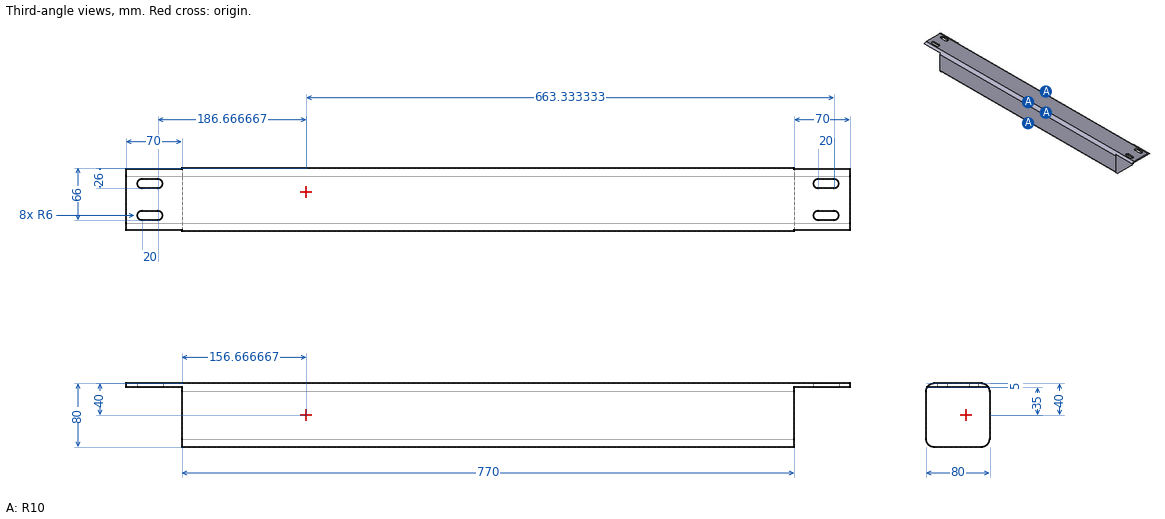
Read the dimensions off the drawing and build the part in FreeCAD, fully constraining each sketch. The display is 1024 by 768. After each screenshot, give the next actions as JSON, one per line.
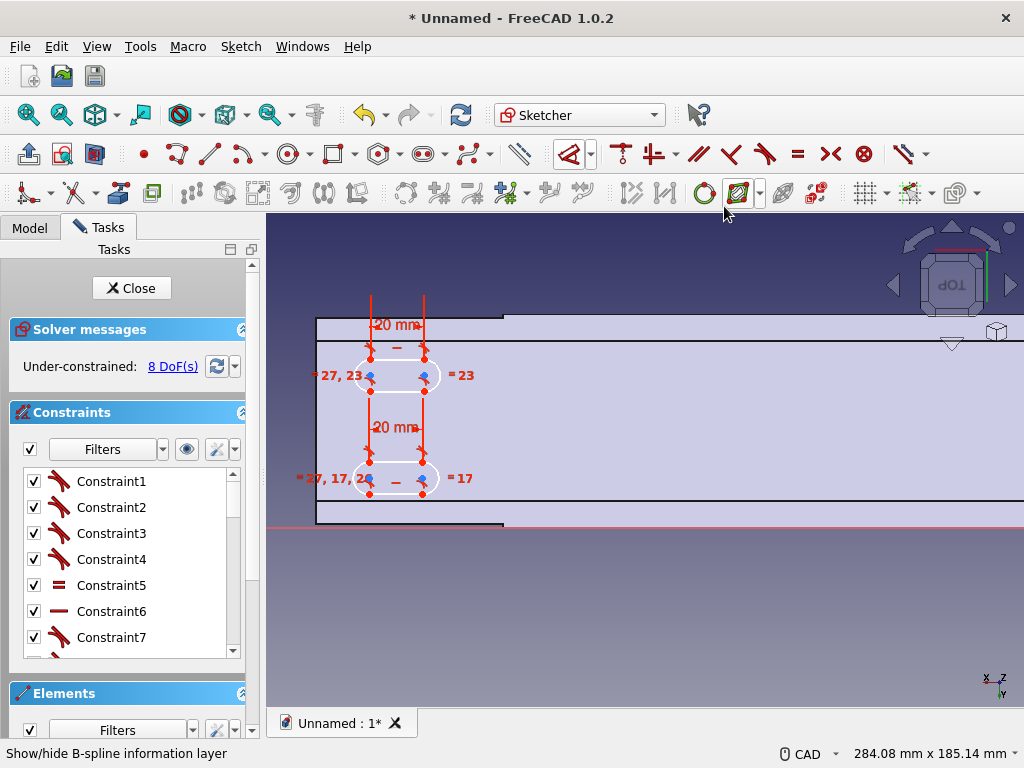
{"action": "scroll", "coordinate": [388, 464], "scroll_direction": "down", "scroll_amount": 9}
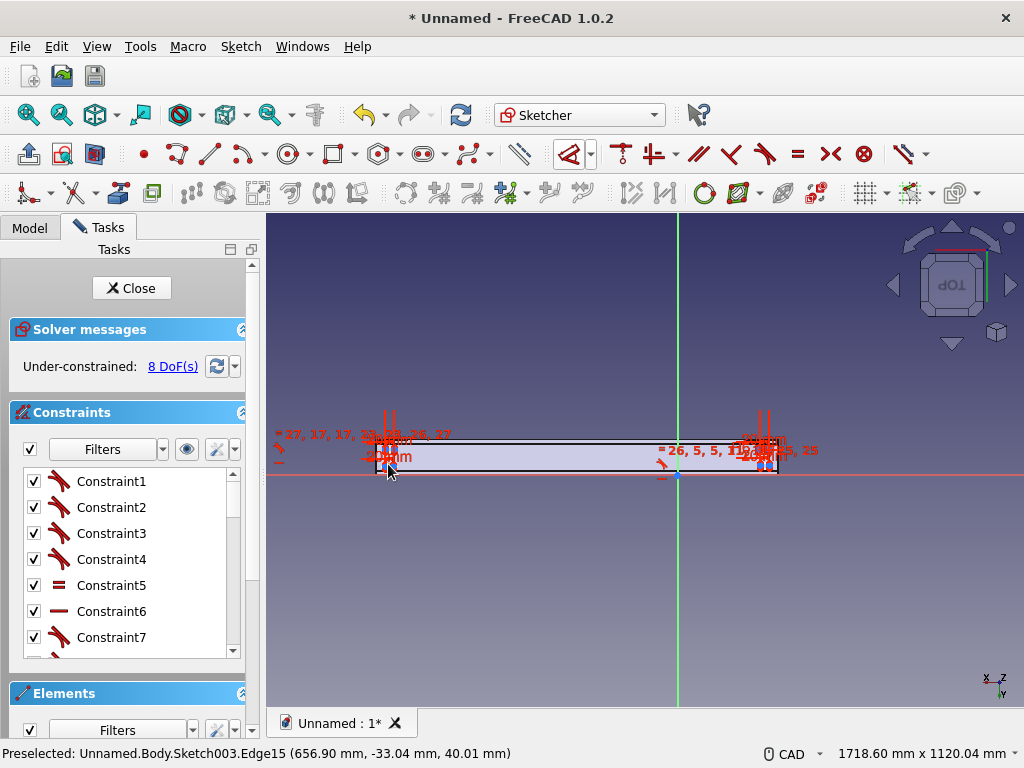
{"action": "scroll", "coordinate": [760, 447], "scroll_direction": "up", "scroll_amount": 8}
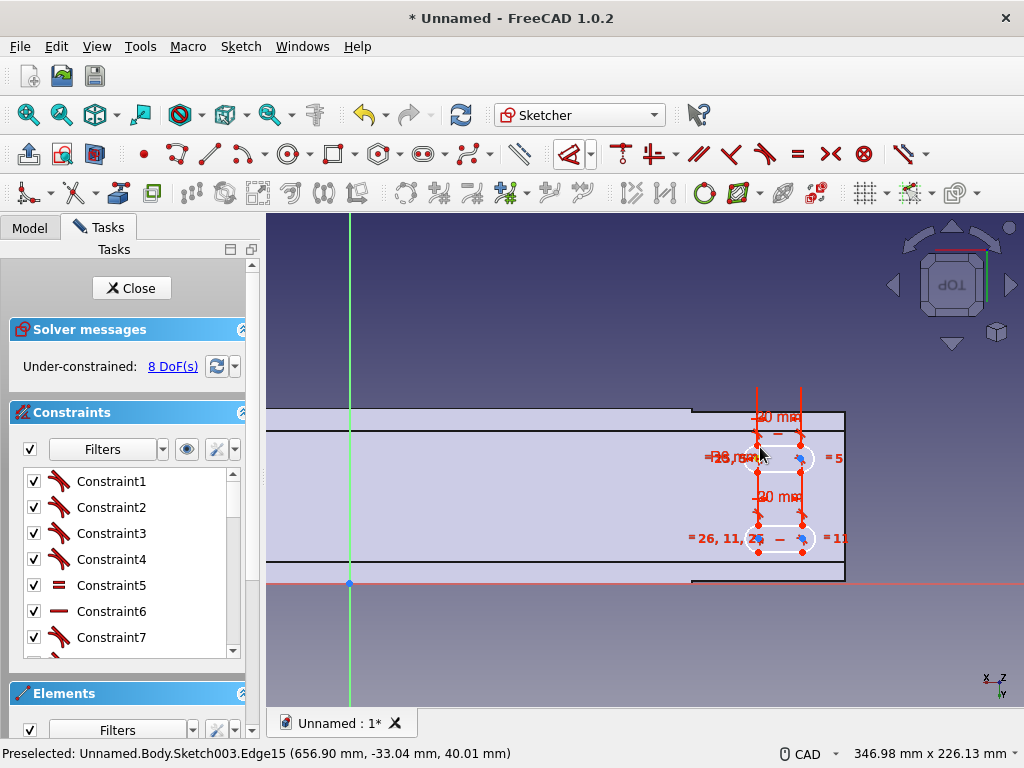
{"action": "left_click", "coordinate": [757, 446]}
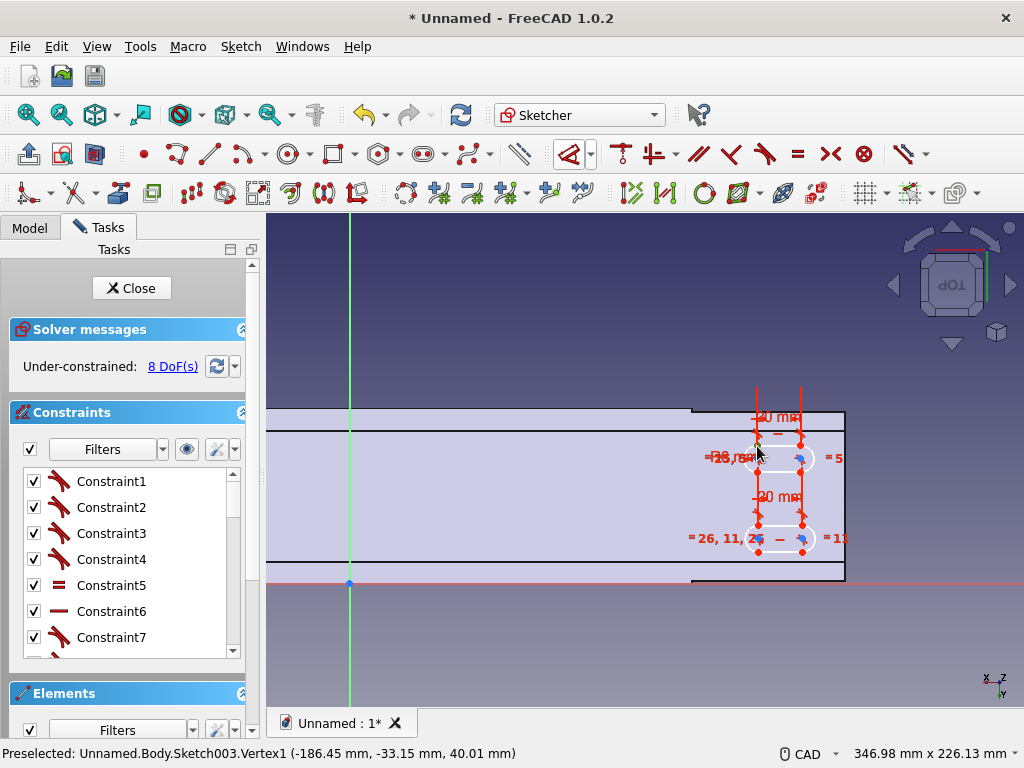
{"action": "key", "text": "i"}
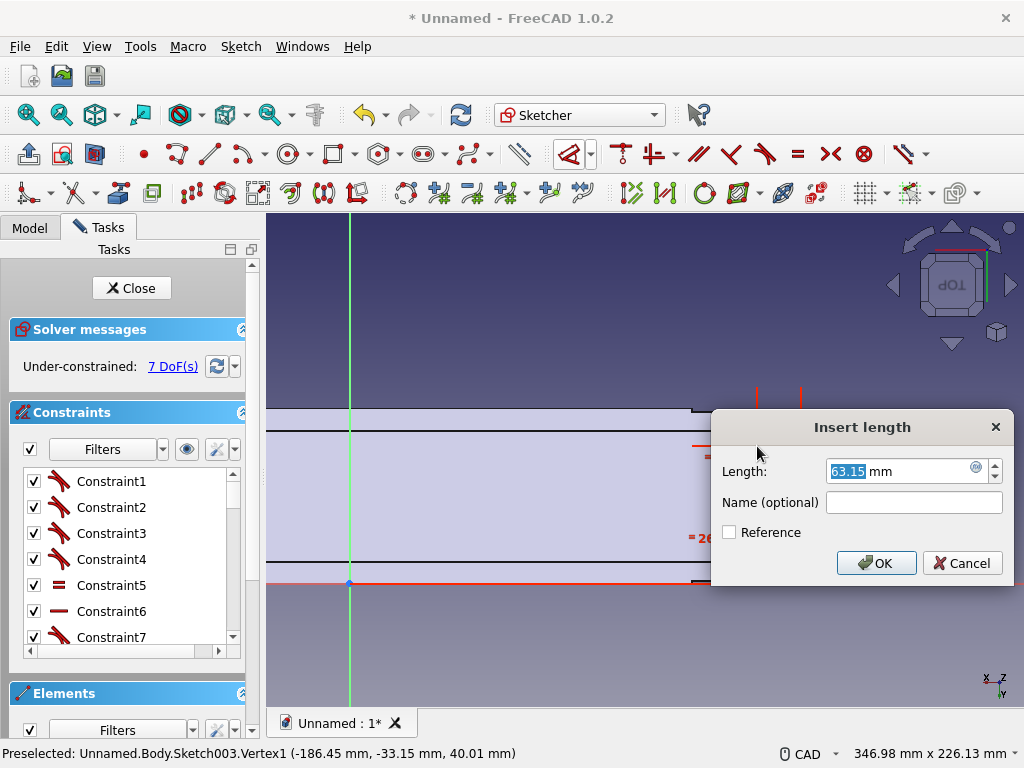
{"action": "type", "text": "66"}
{"action": "key", "text": "Return"}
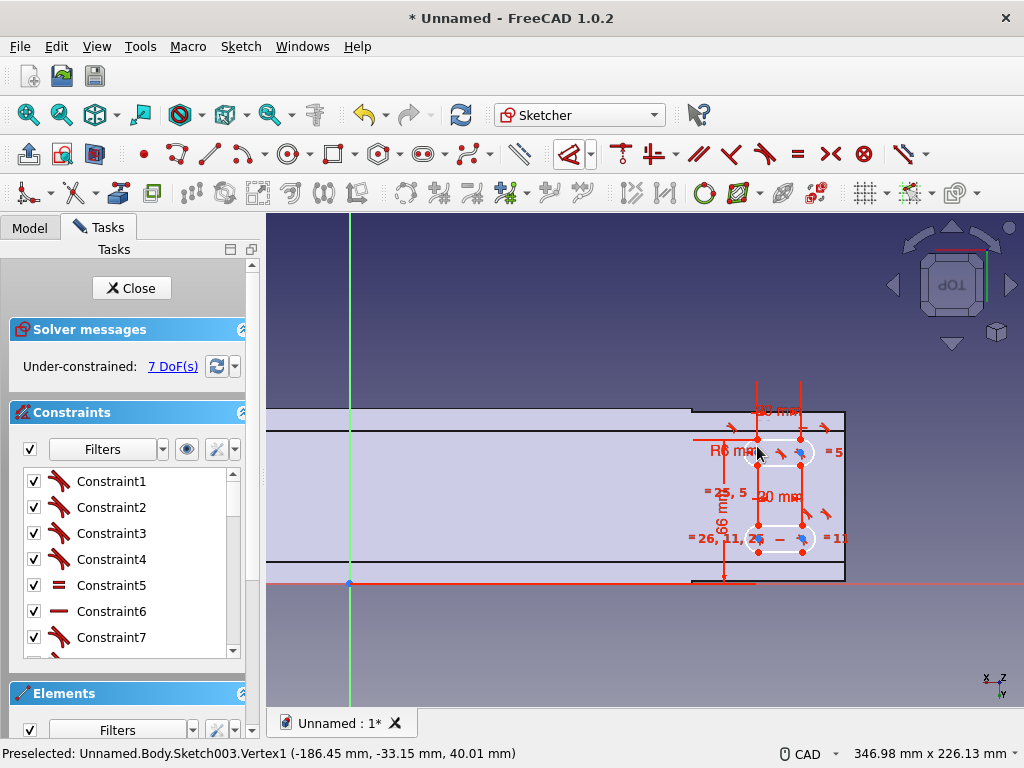
{"action": "left_click", "coordinate": [758, 526]}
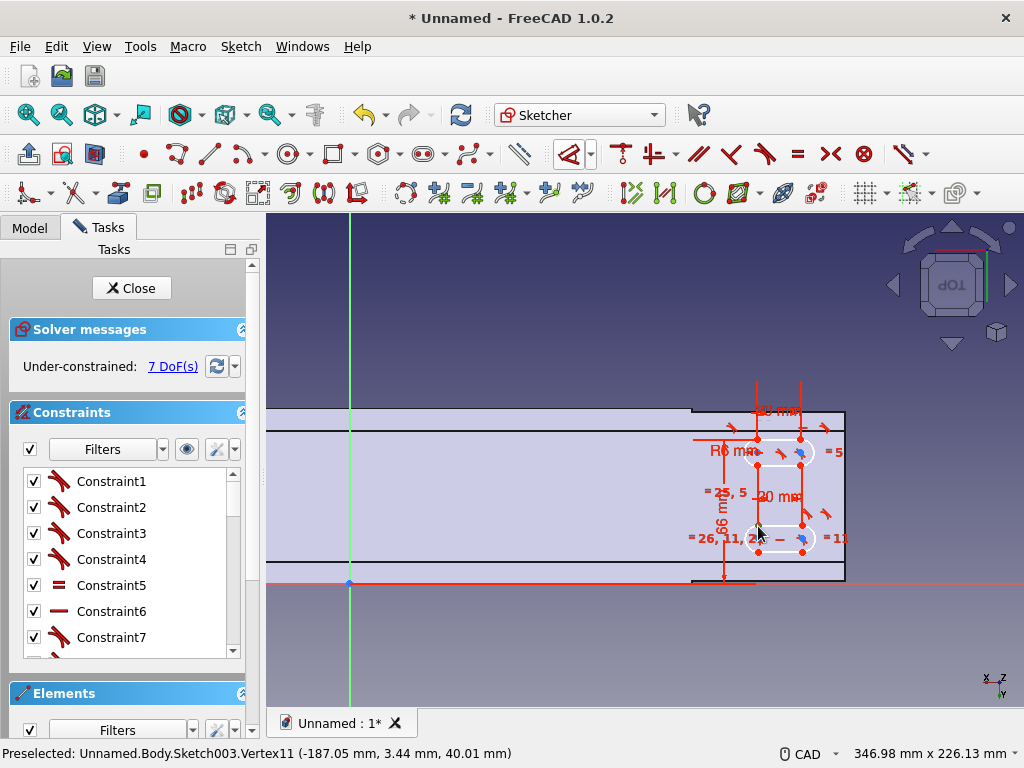
{"action": "left_click", "coordinate": [590, 154]}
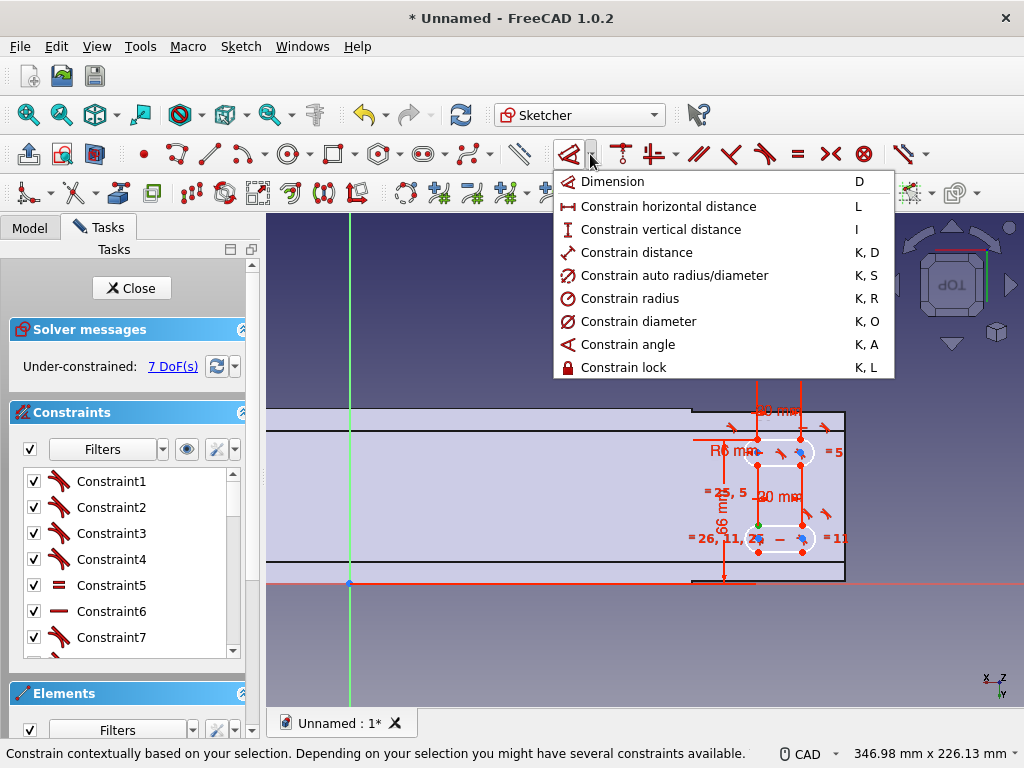
{"action": "left_click", "coordinate": [724, 230]}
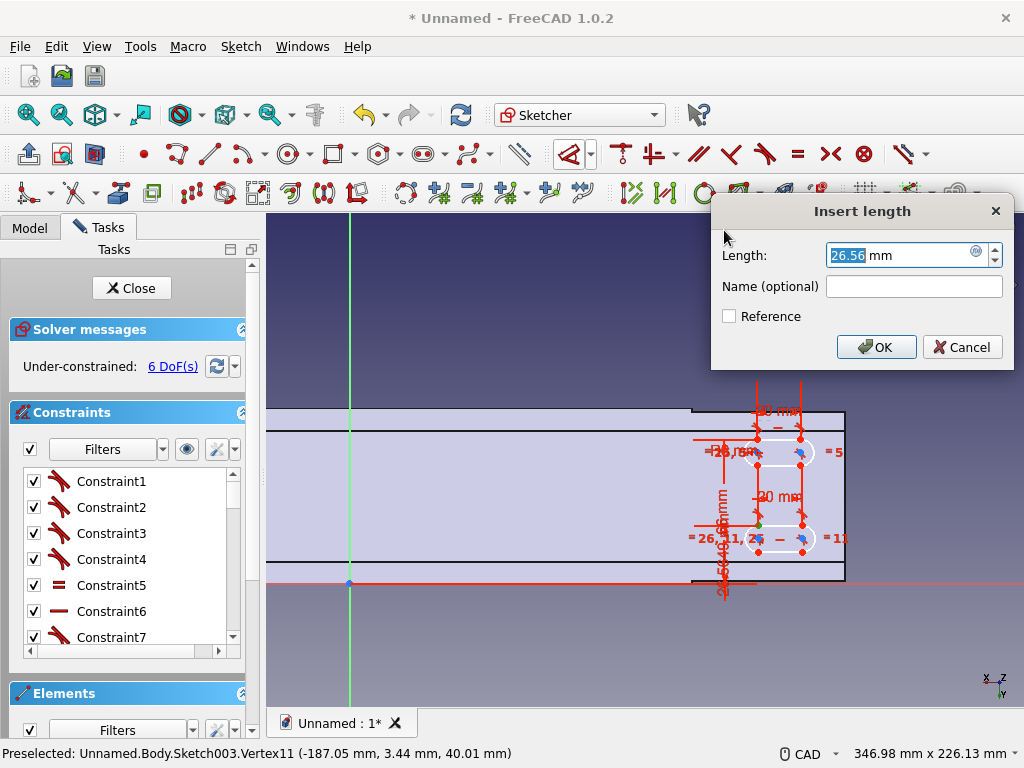
{"action": "type", "text": "26"}
{"action": "key", "text": "Return"}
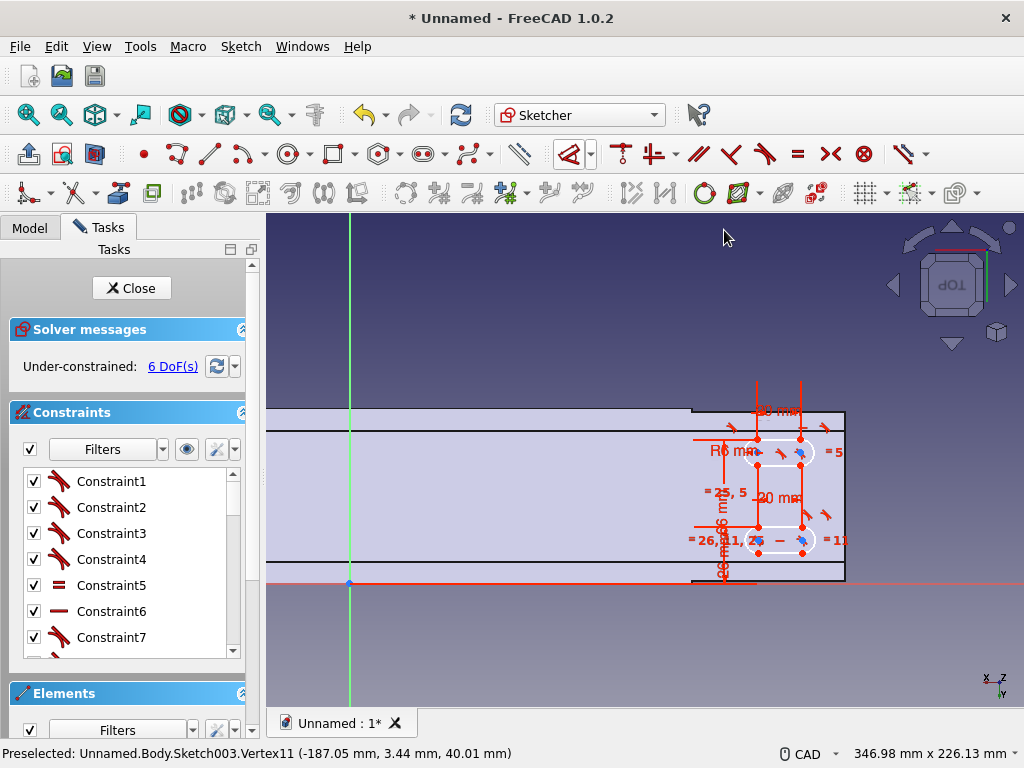
{"action": "scroll", "coordinate": [760, 447], "scroll_direction": "down", "scroll_amount": 8}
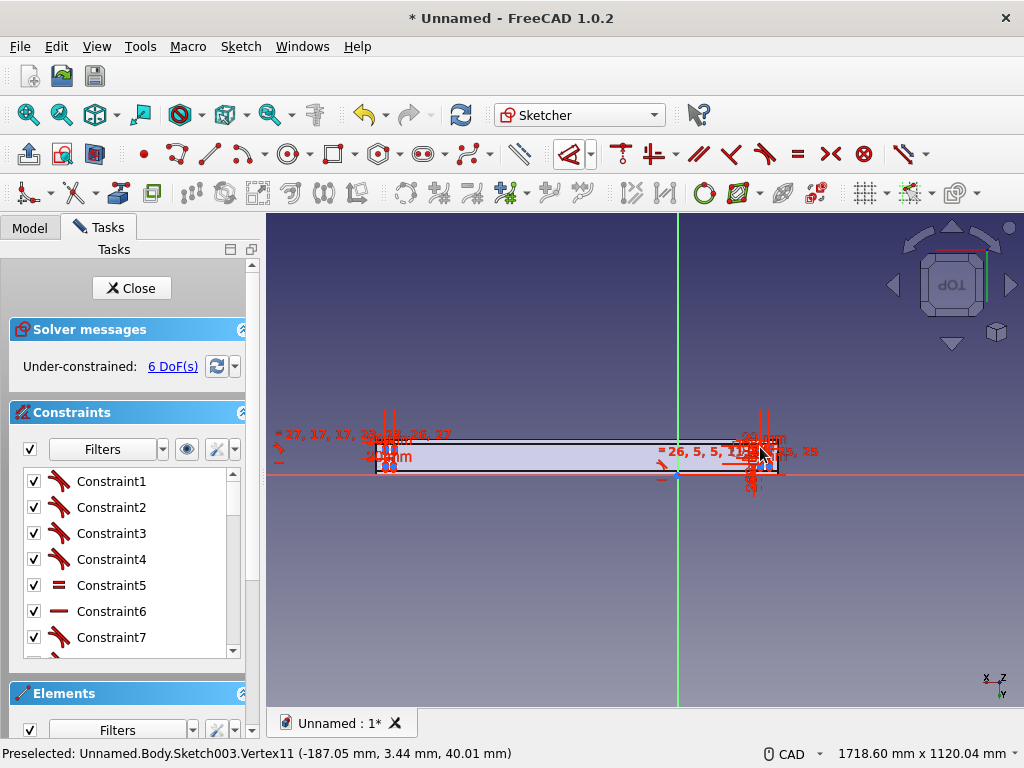
{"action": "scroll", "coordinate": [385, 464], "scroll_direction": "up", "scroll_amount": 8}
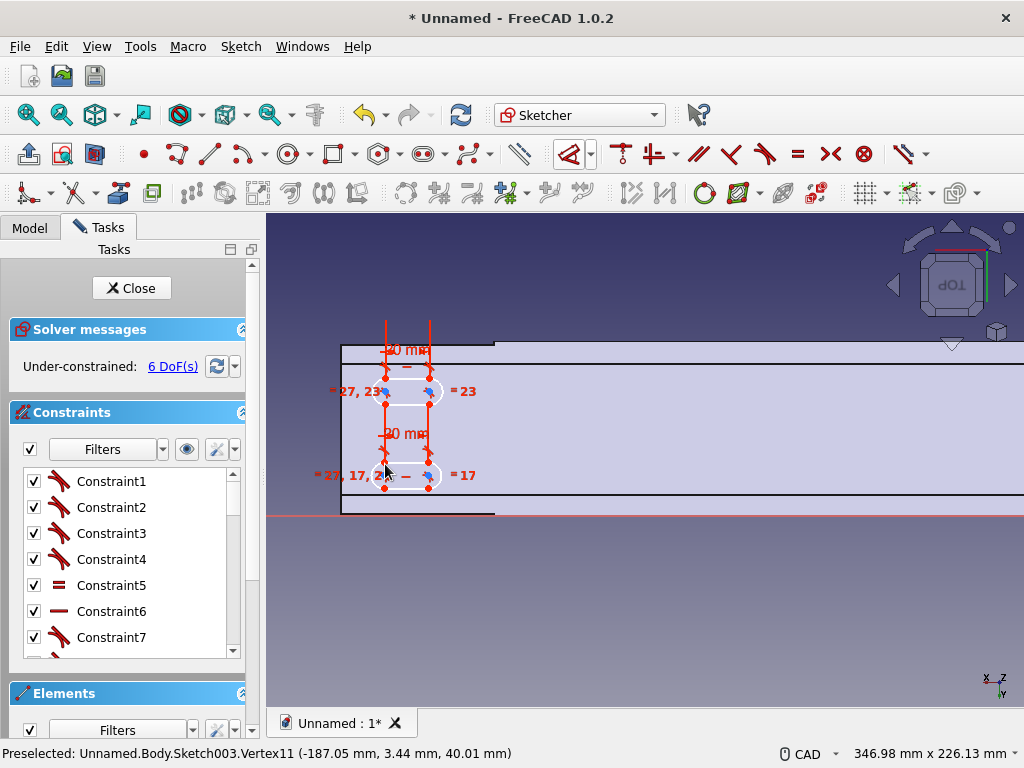
{"action": "left_click", "coordinate": [385, 463]}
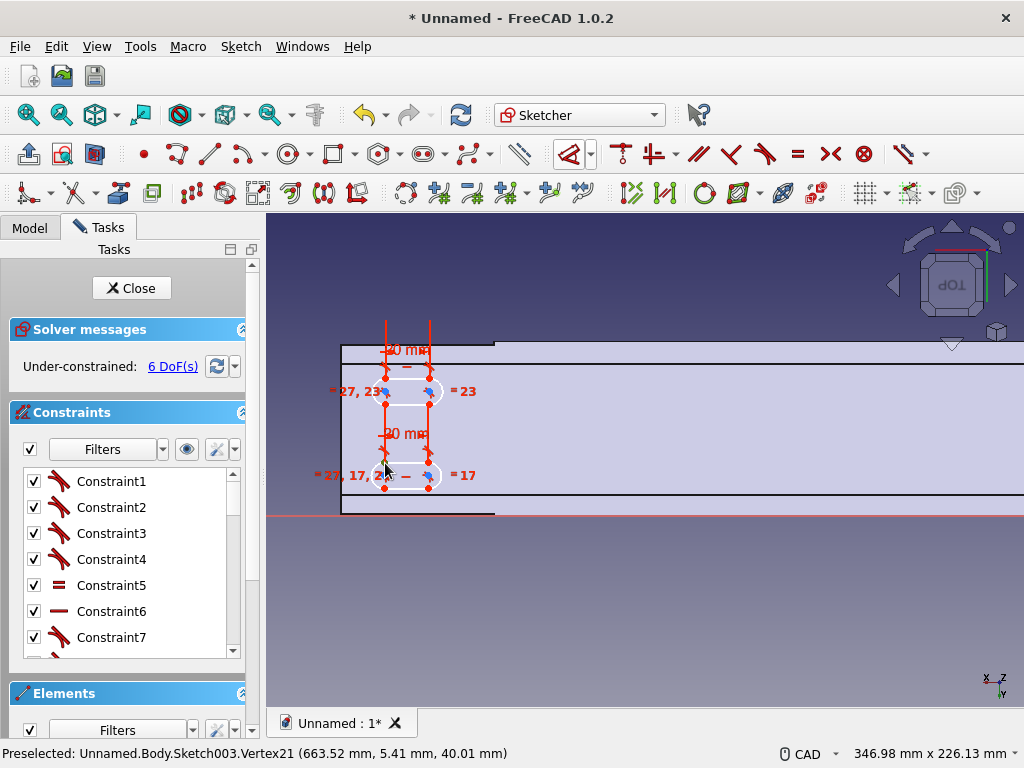
{"action": "key", "text": "i"}